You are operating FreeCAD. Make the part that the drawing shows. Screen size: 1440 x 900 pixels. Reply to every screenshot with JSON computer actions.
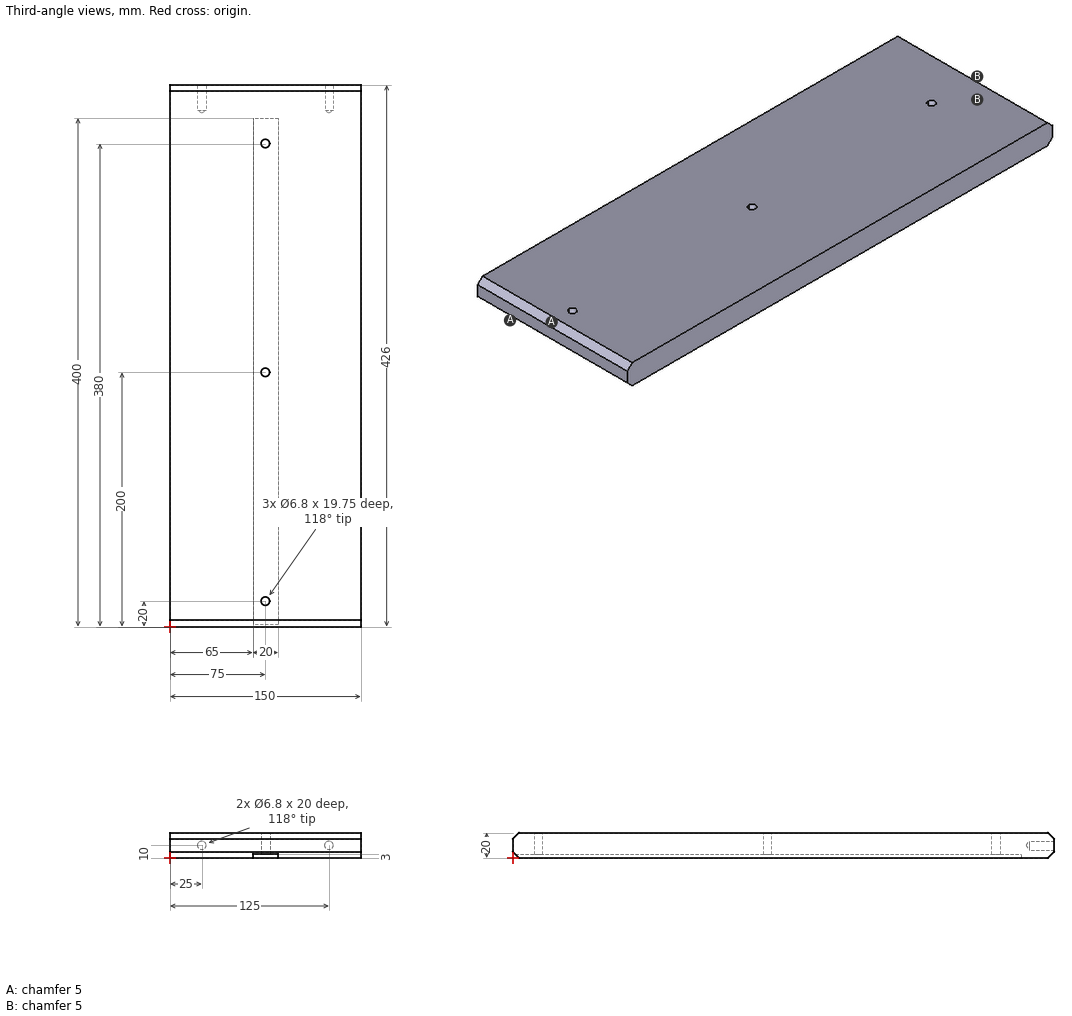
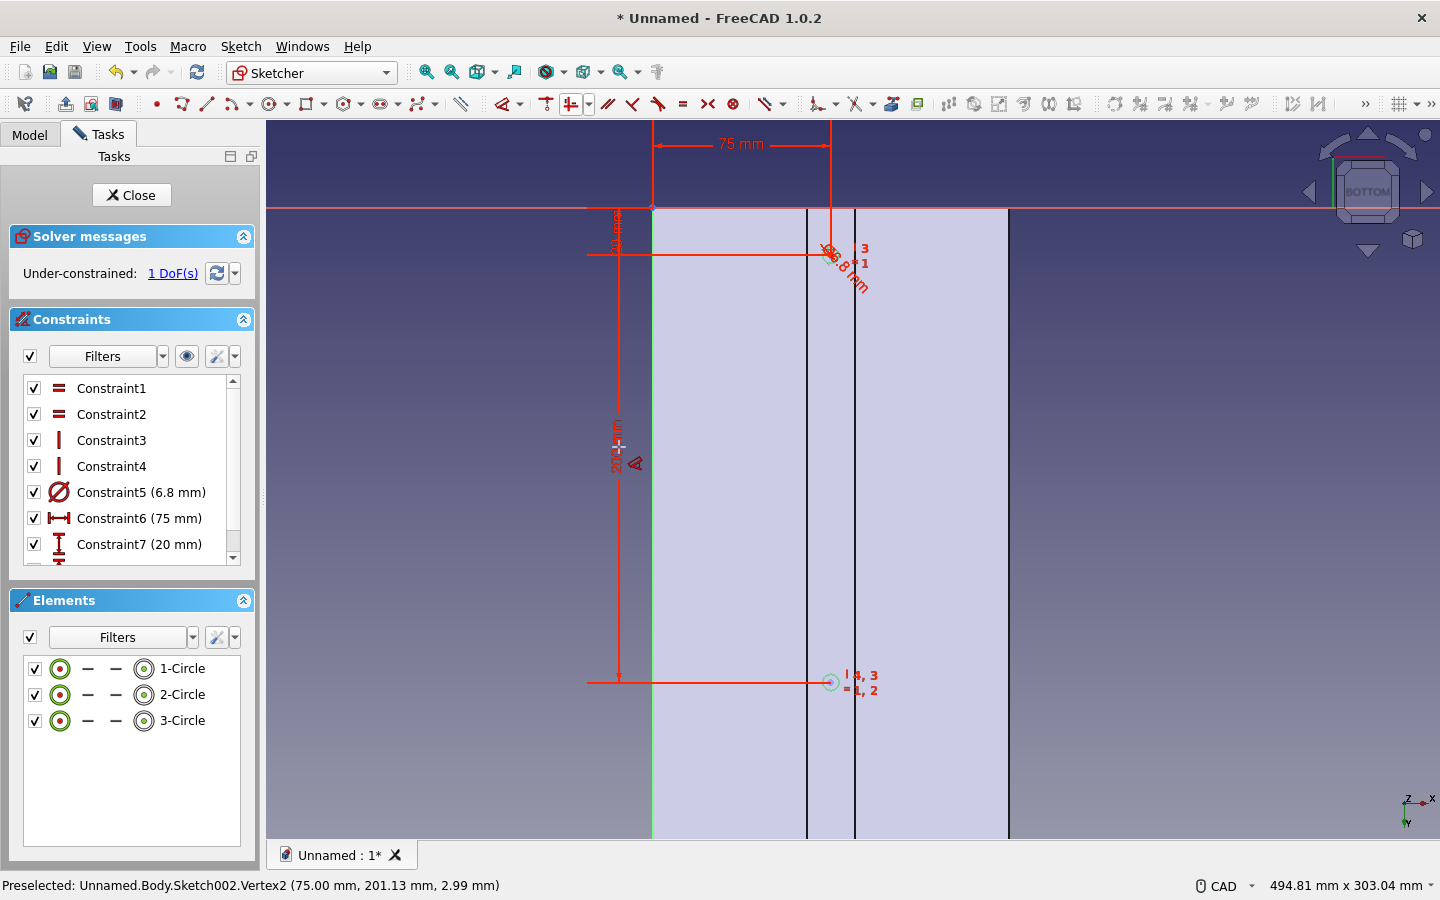
{"action": "scroll", "coordinate": [831, 257], "scroll_direction": "down", "scroll_amount": 3}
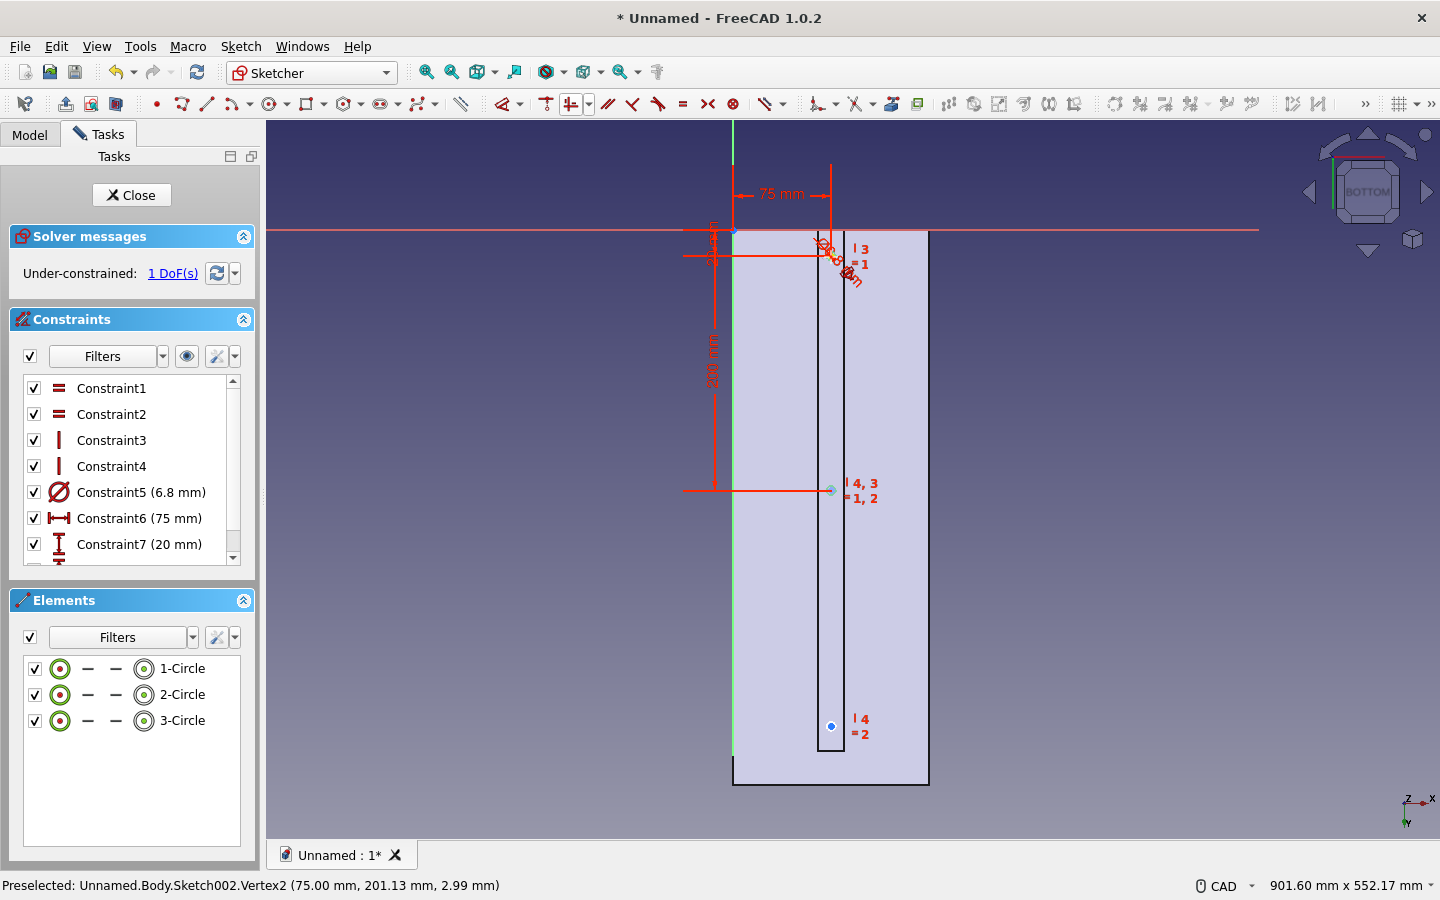
{"action": "left_click", "coordinate": [831, 726]}
{"action": "left_click", "coordinate": [699, 478]}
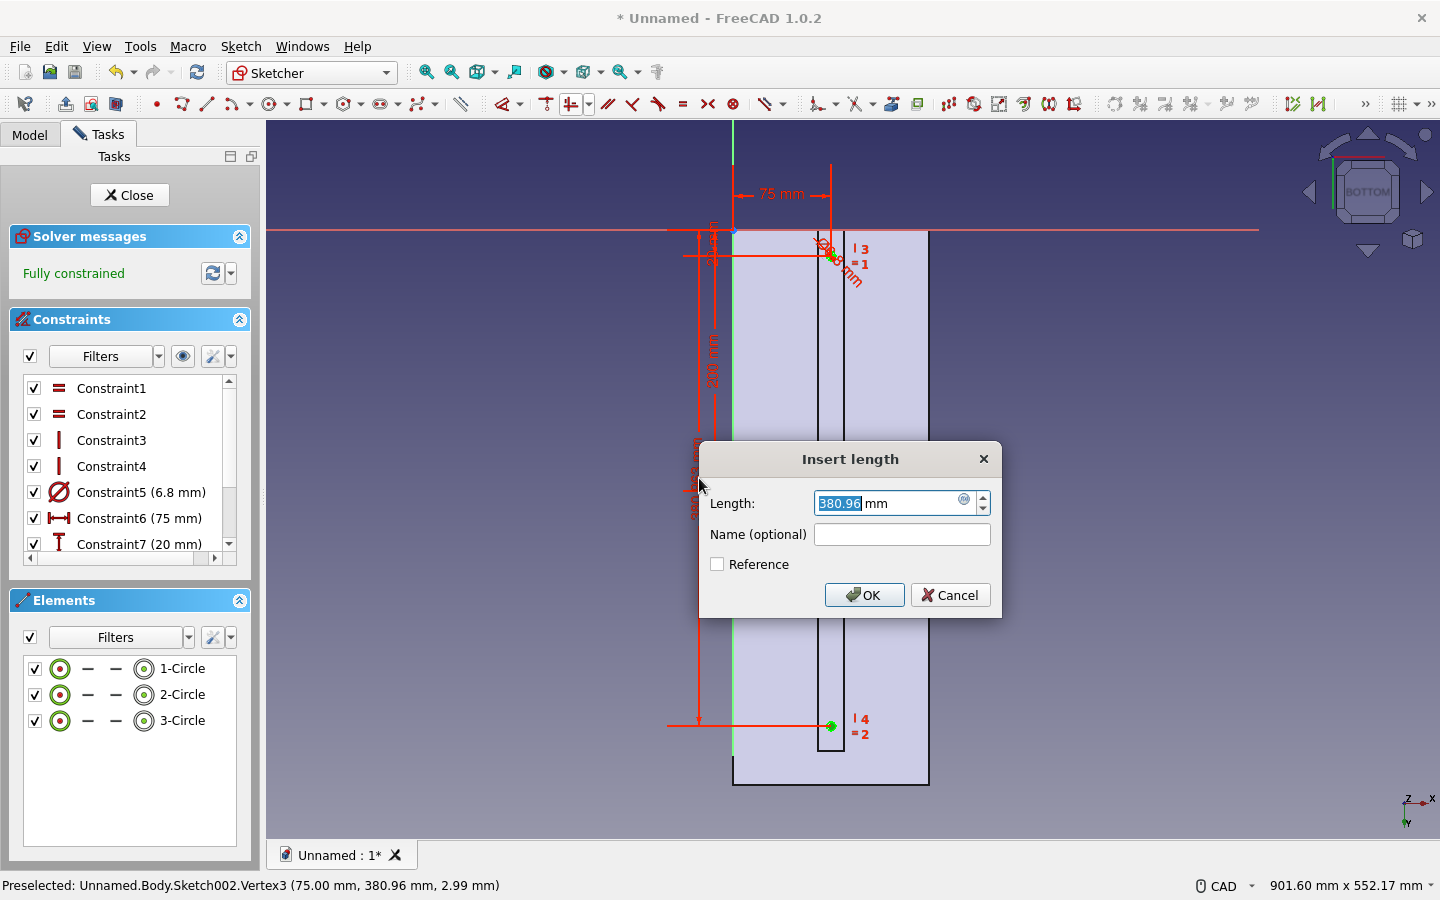
{"action": "type", "text": "380"}
{"action": "key", "text": "Return"}
{"action": "key", "text": "Escape"}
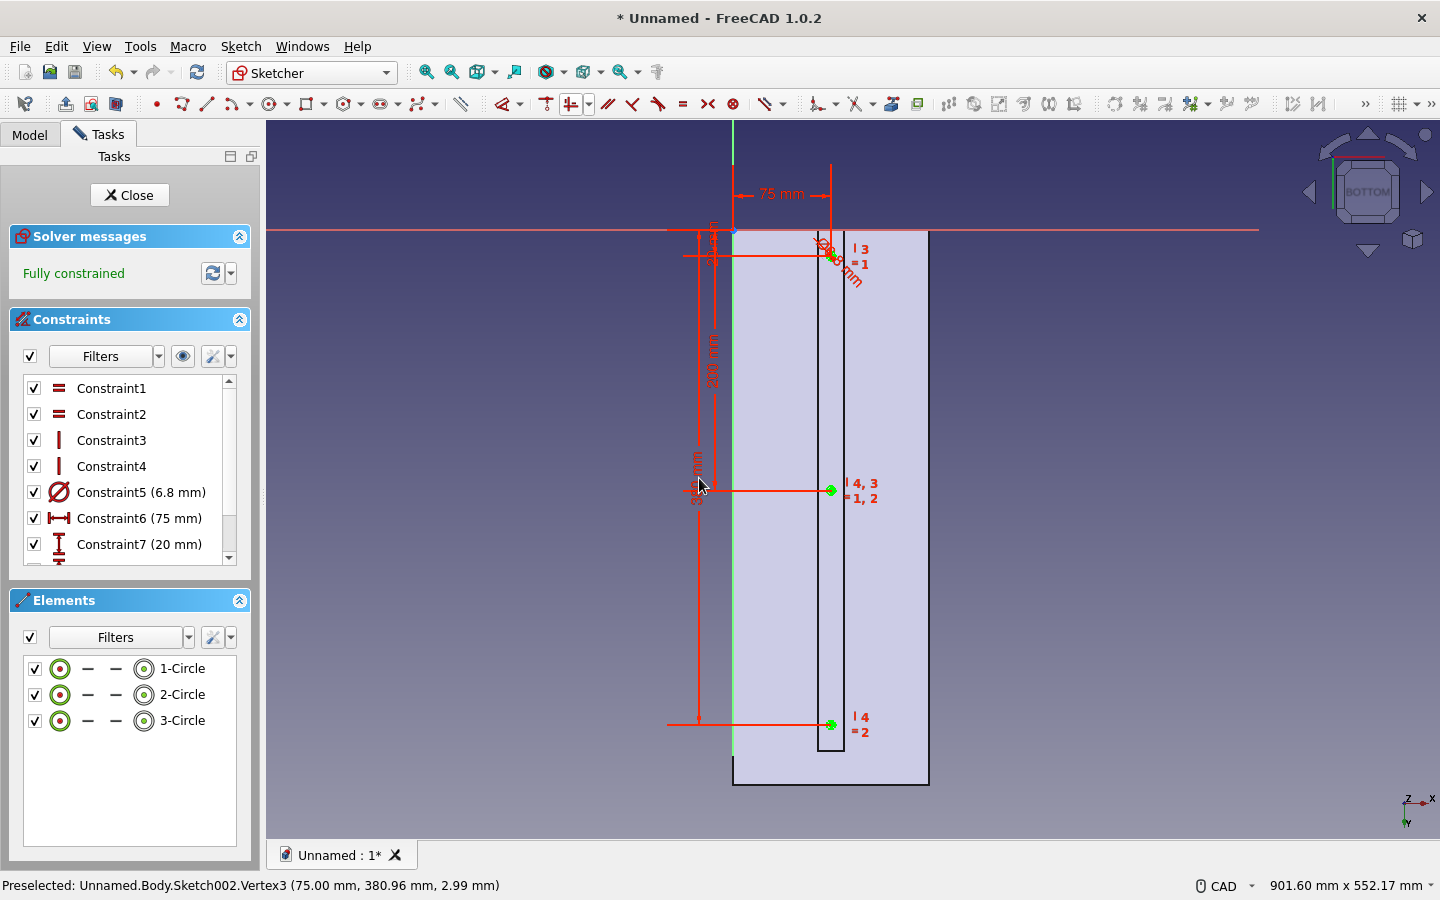
{"action": "left_click", "coordinate": [130, 195]}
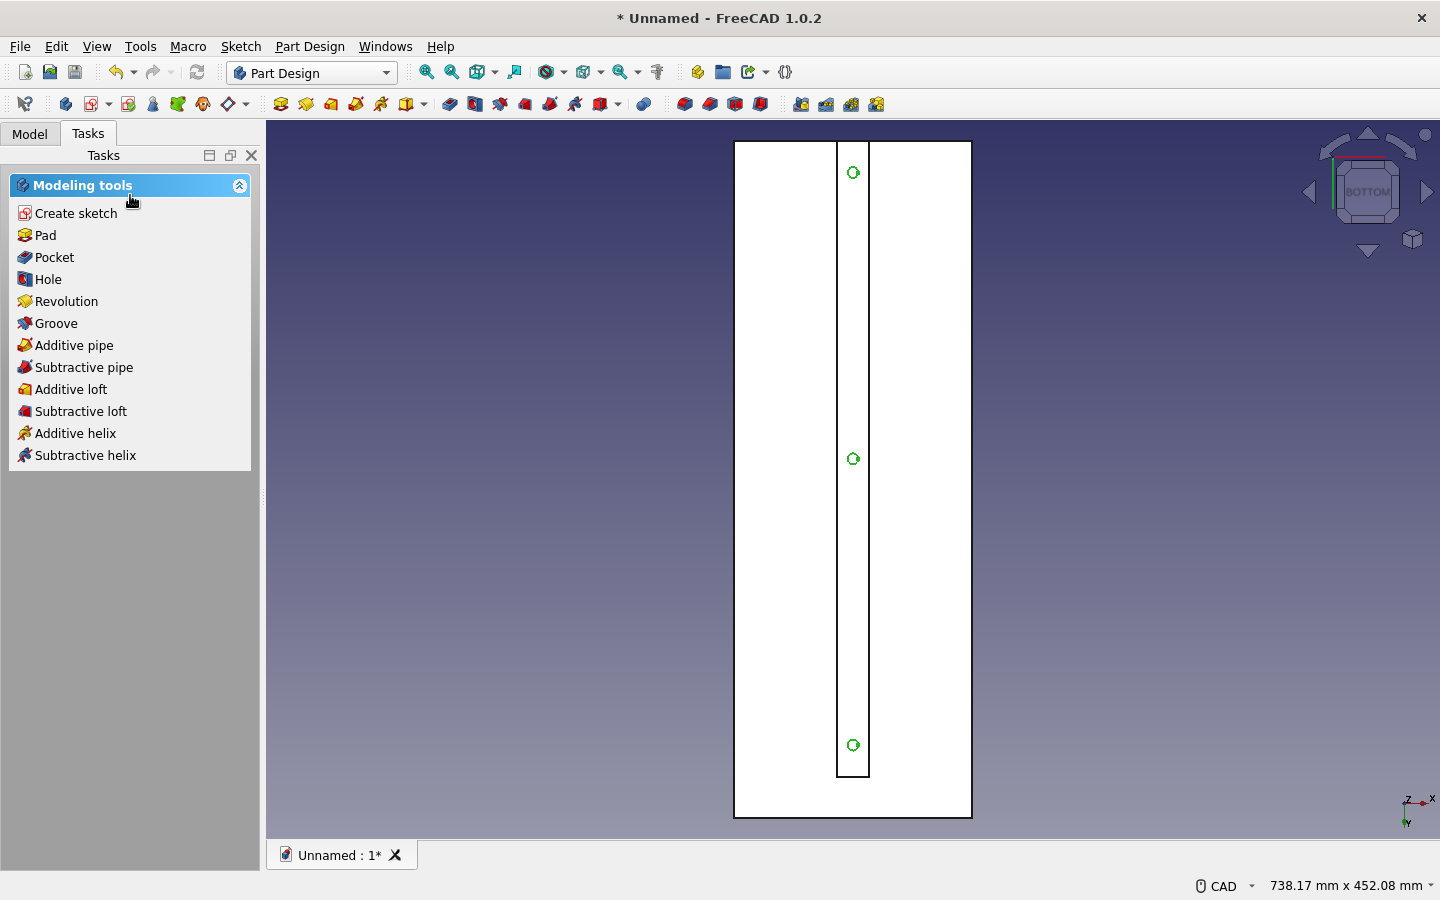
{"action": "left_click", "coordinate": [475, 104]}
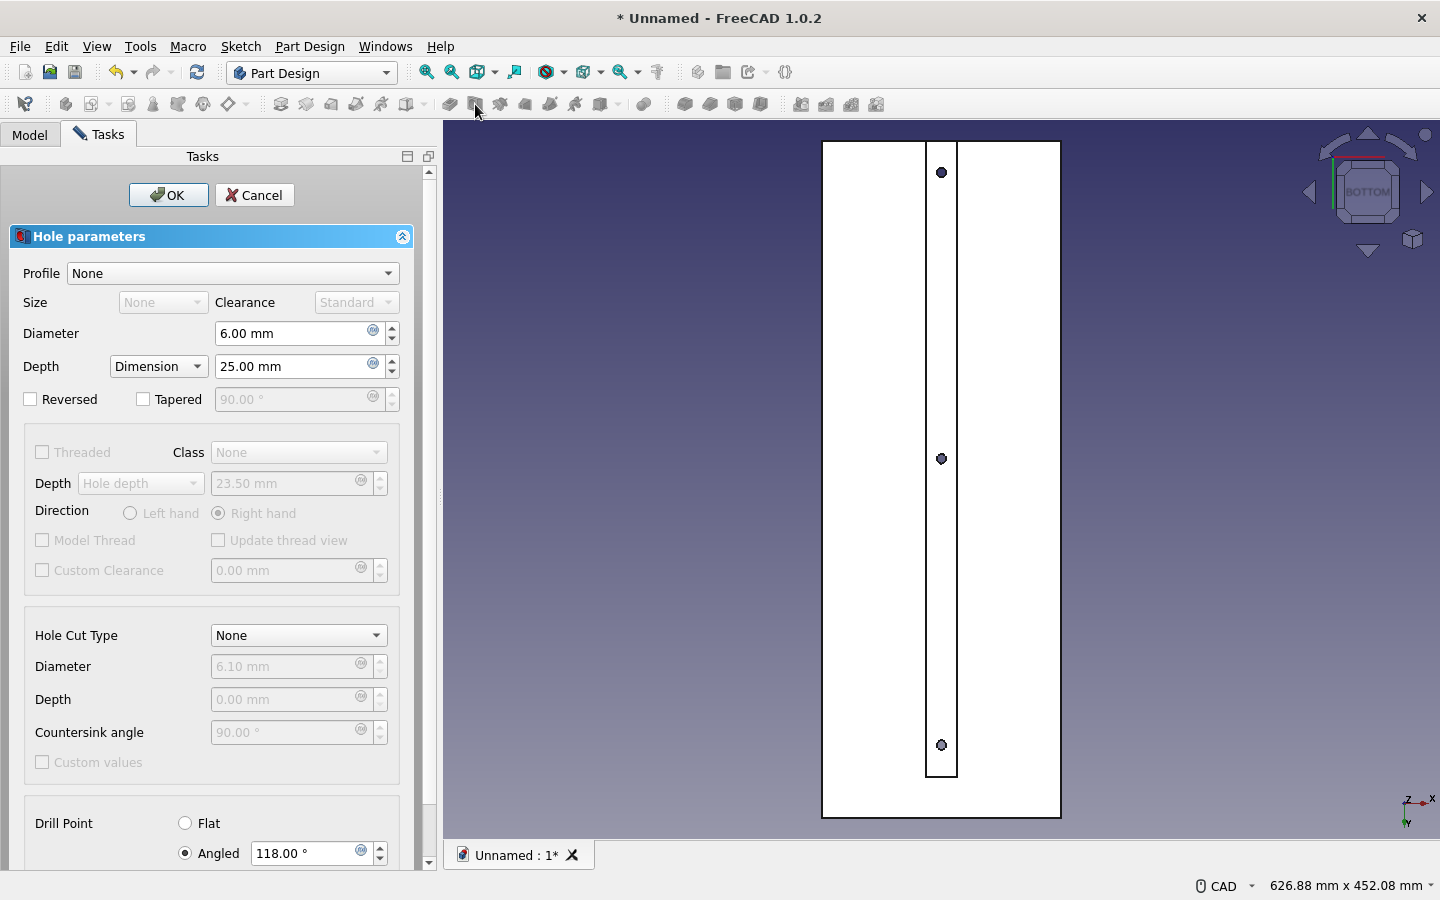
{"action": "triple_click", "coordinate": [300, 334]}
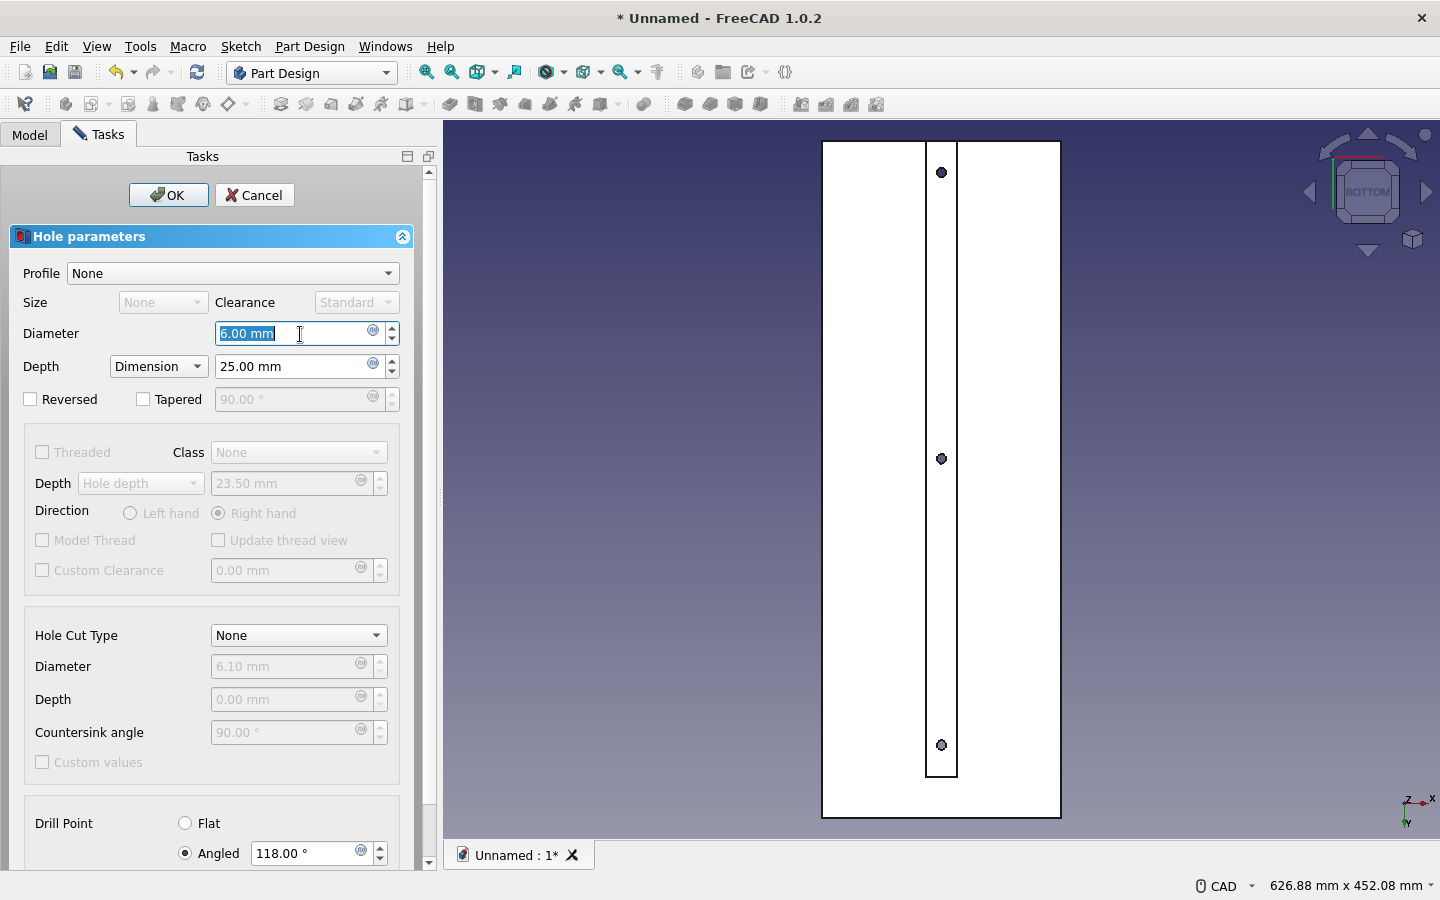
{"action": "type", "text": "6.8"}
{"action": "key", "text": "Tab"}